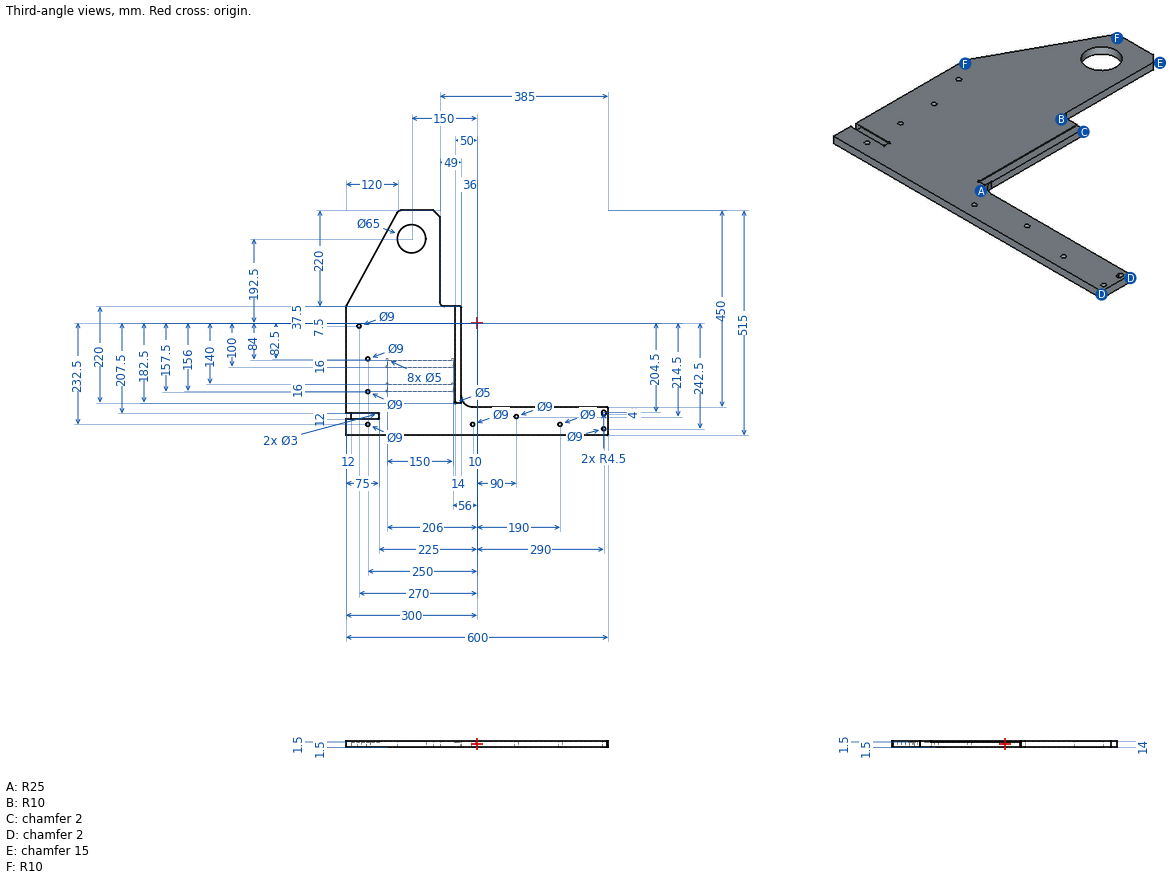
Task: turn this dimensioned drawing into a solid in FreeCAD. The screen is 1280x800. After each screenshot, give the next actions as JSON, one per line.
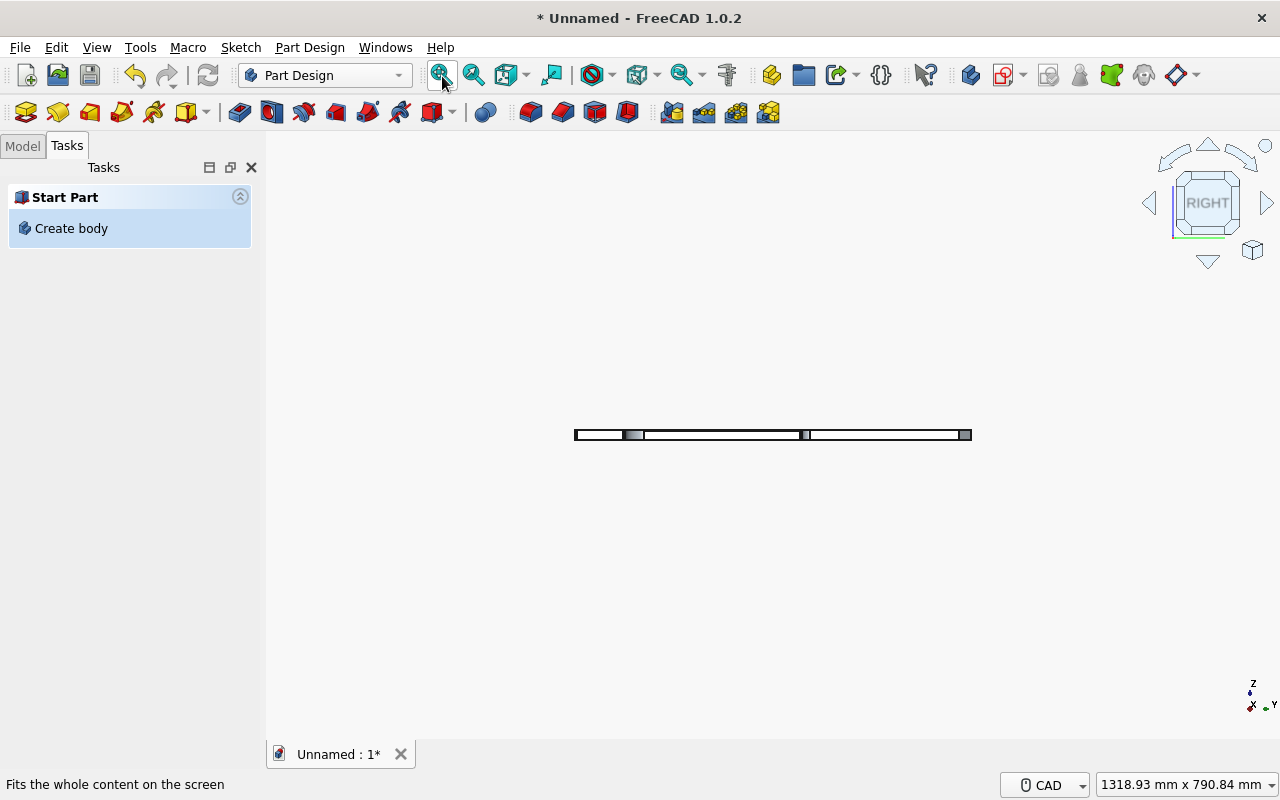
{"action": "key", "text": "5"}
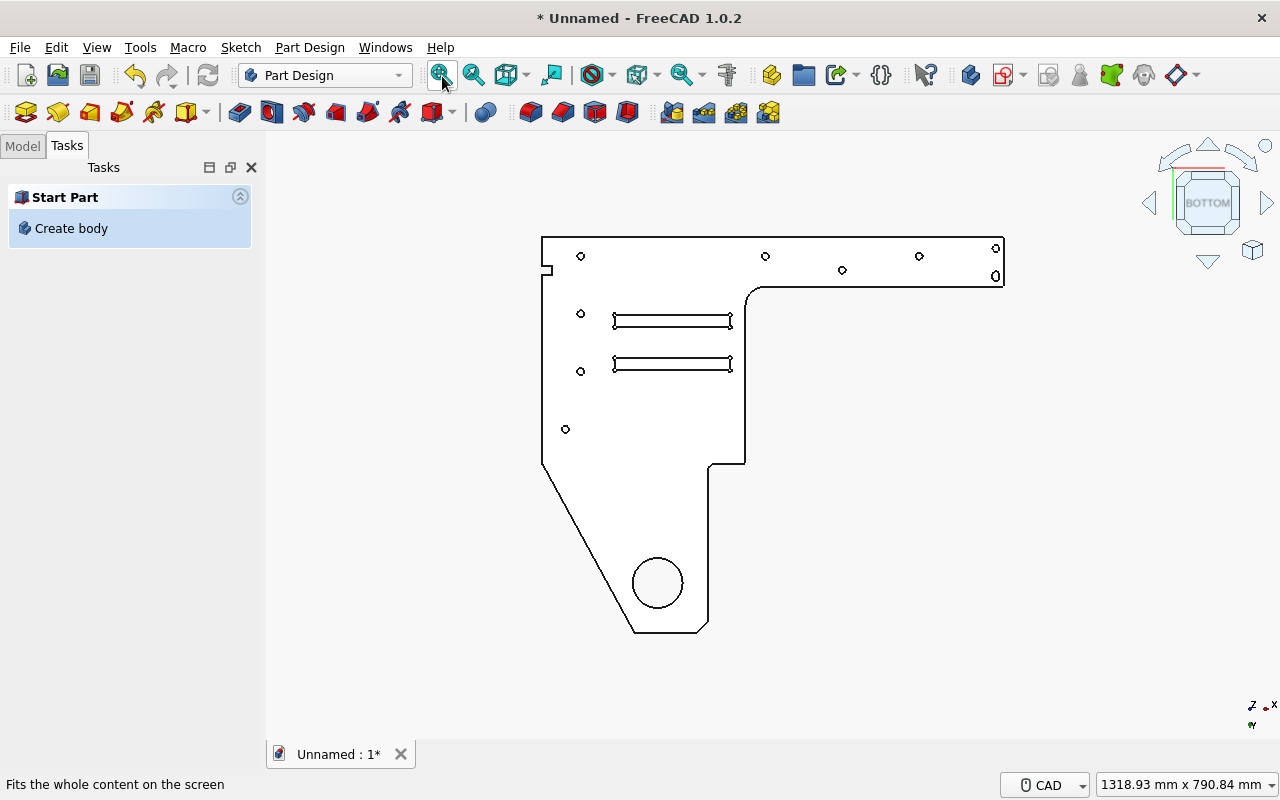
{"action": "scroll", "coordinate": [635, 632], "scroll_direction": "up", "scroll_amount": 7}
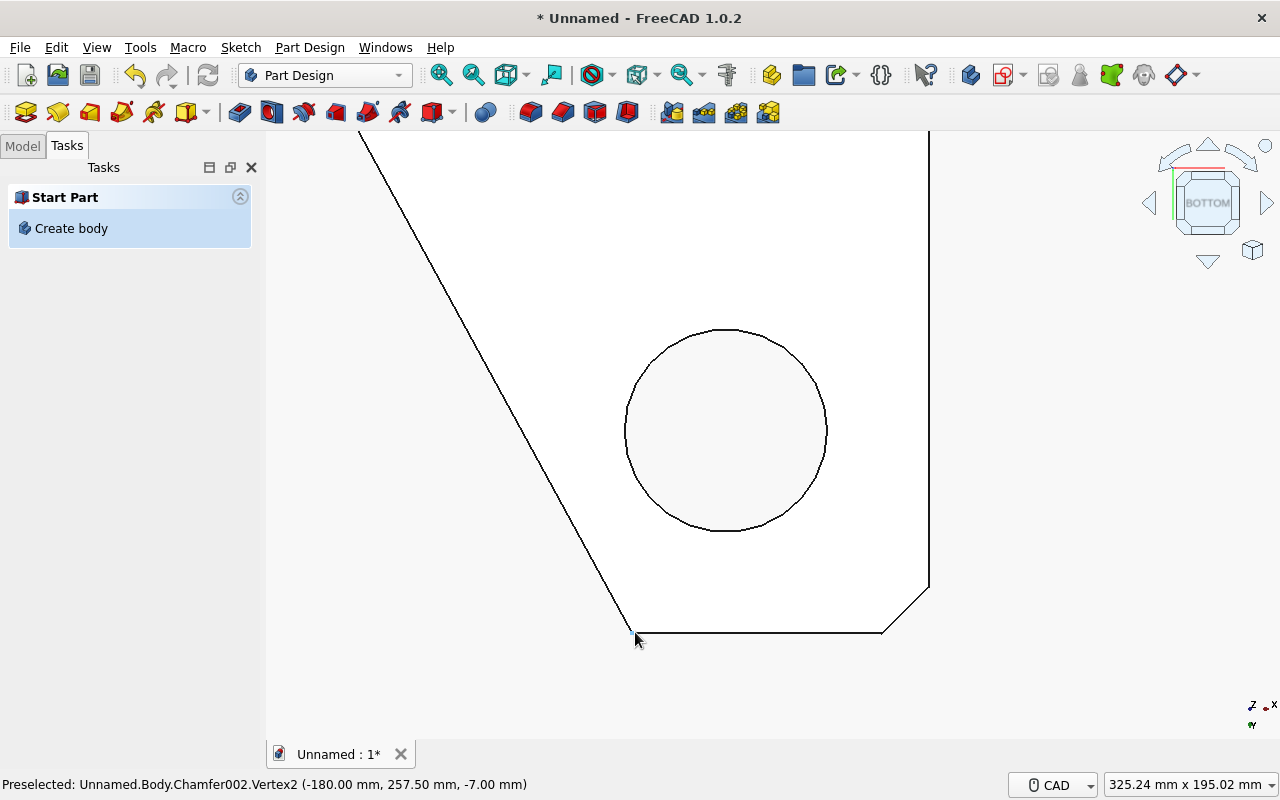
{"action": "left_click", "coordinate": [442, 76]}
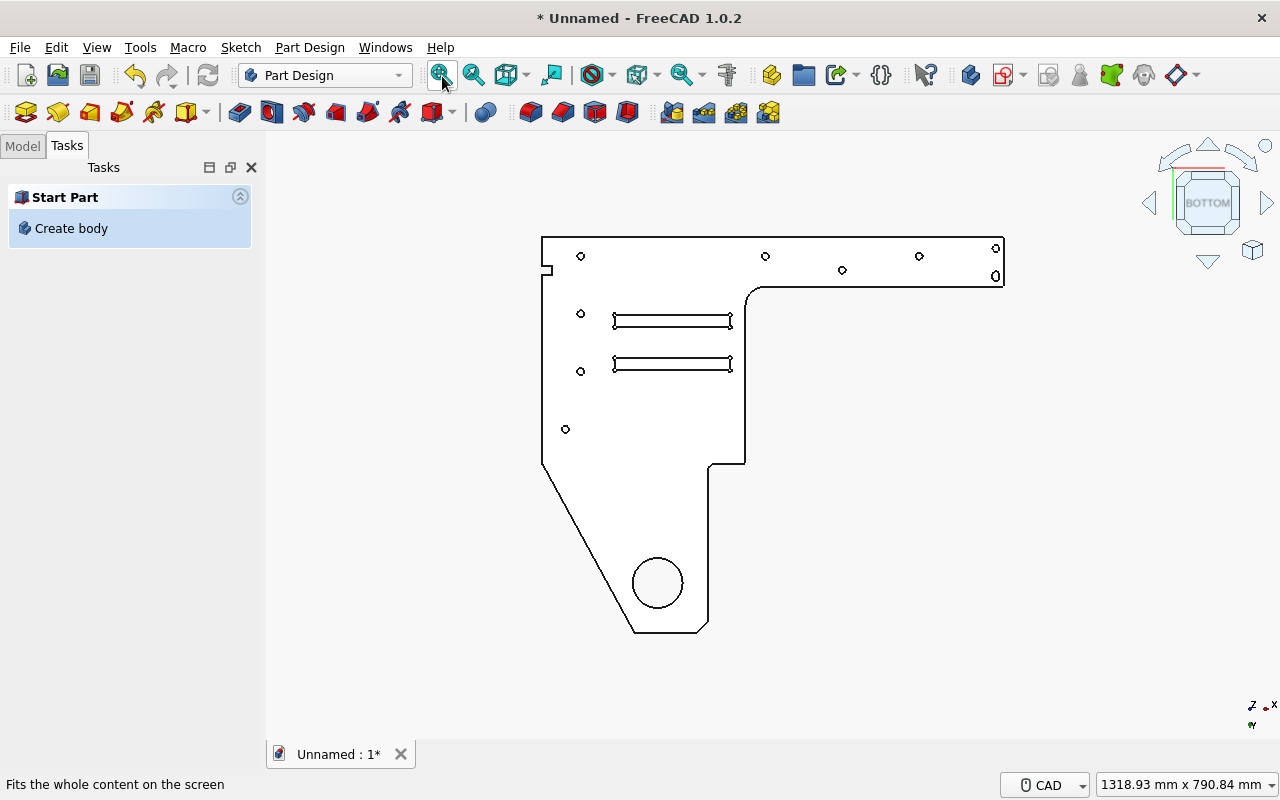
{"action": "key", "text": "4"}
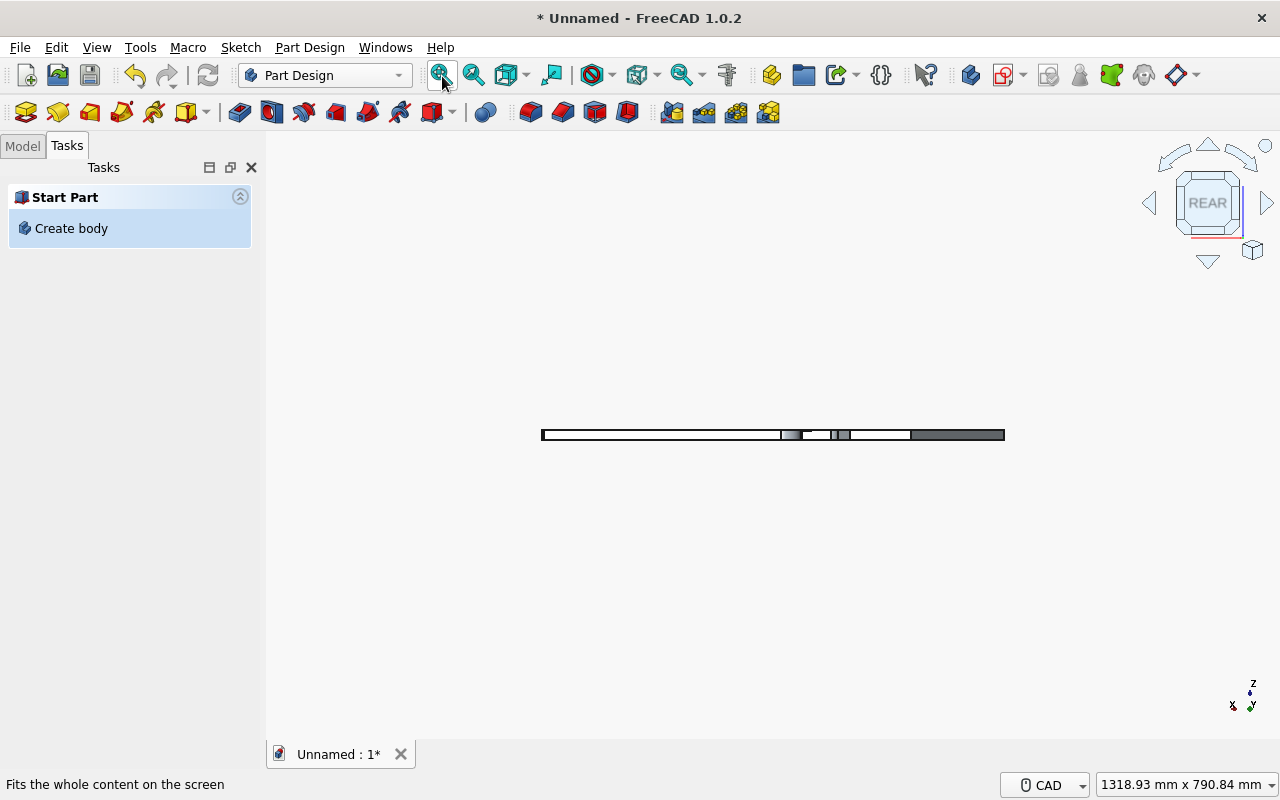
{"action": "scroll", "coordinate": [911, 434], "scroll_direction": "up", "scroll_amount": 7}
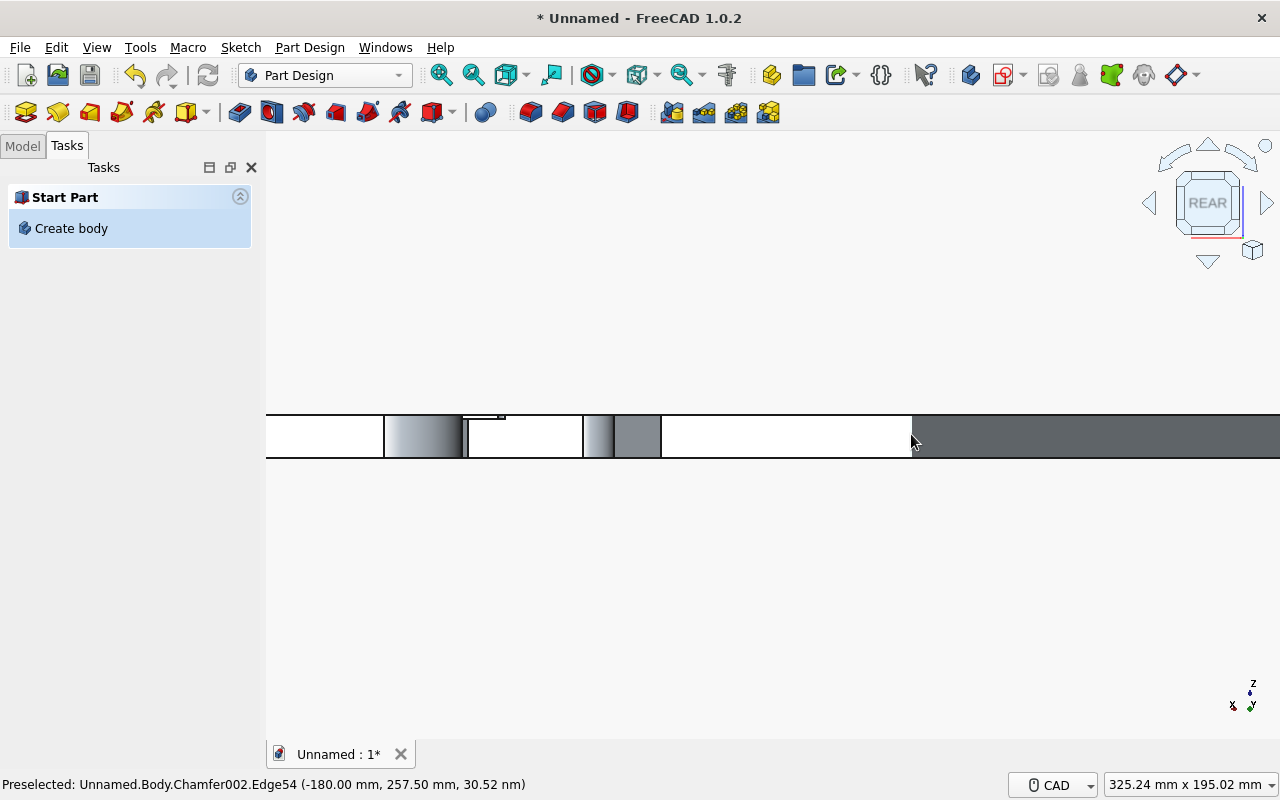
{"action": "left_click", "coordinate": [911, 436]}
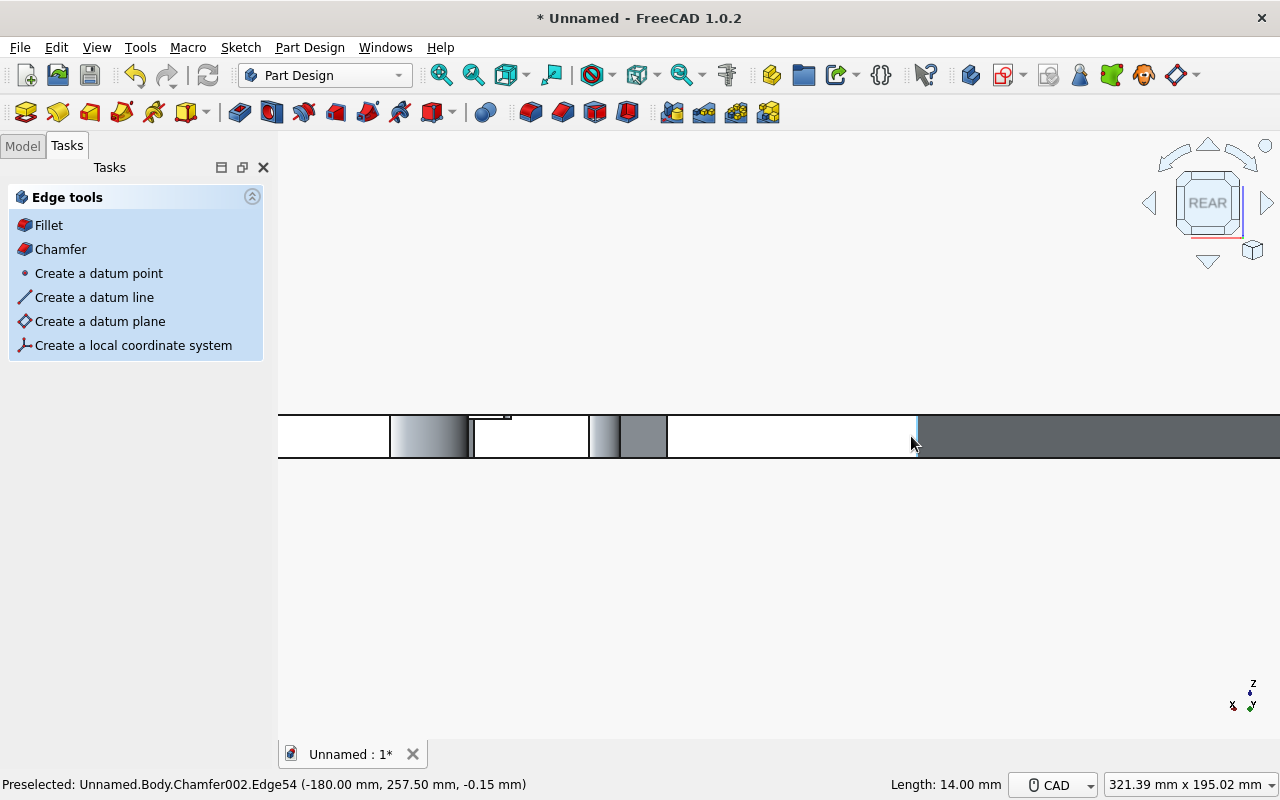
{"action": "left_click", "coordinate": [442, 76]}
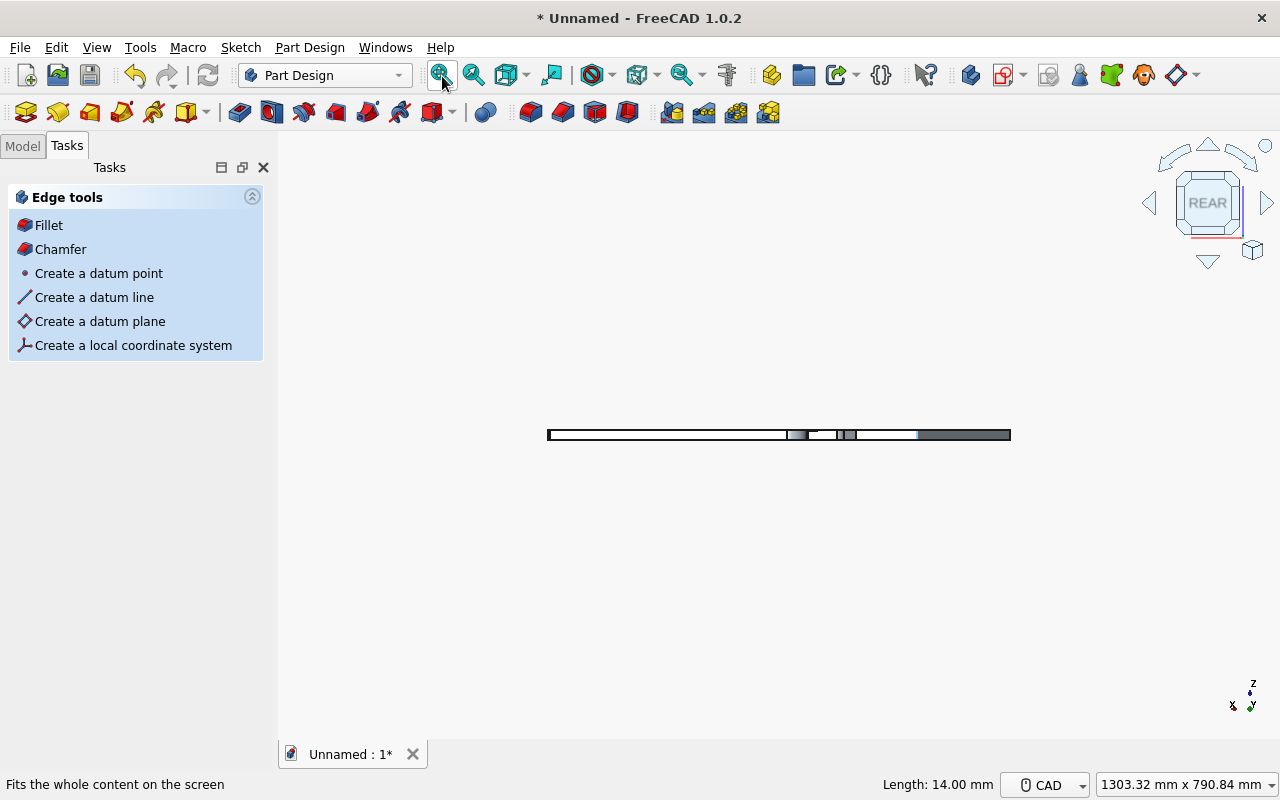
{"action": "key", "text": "6"}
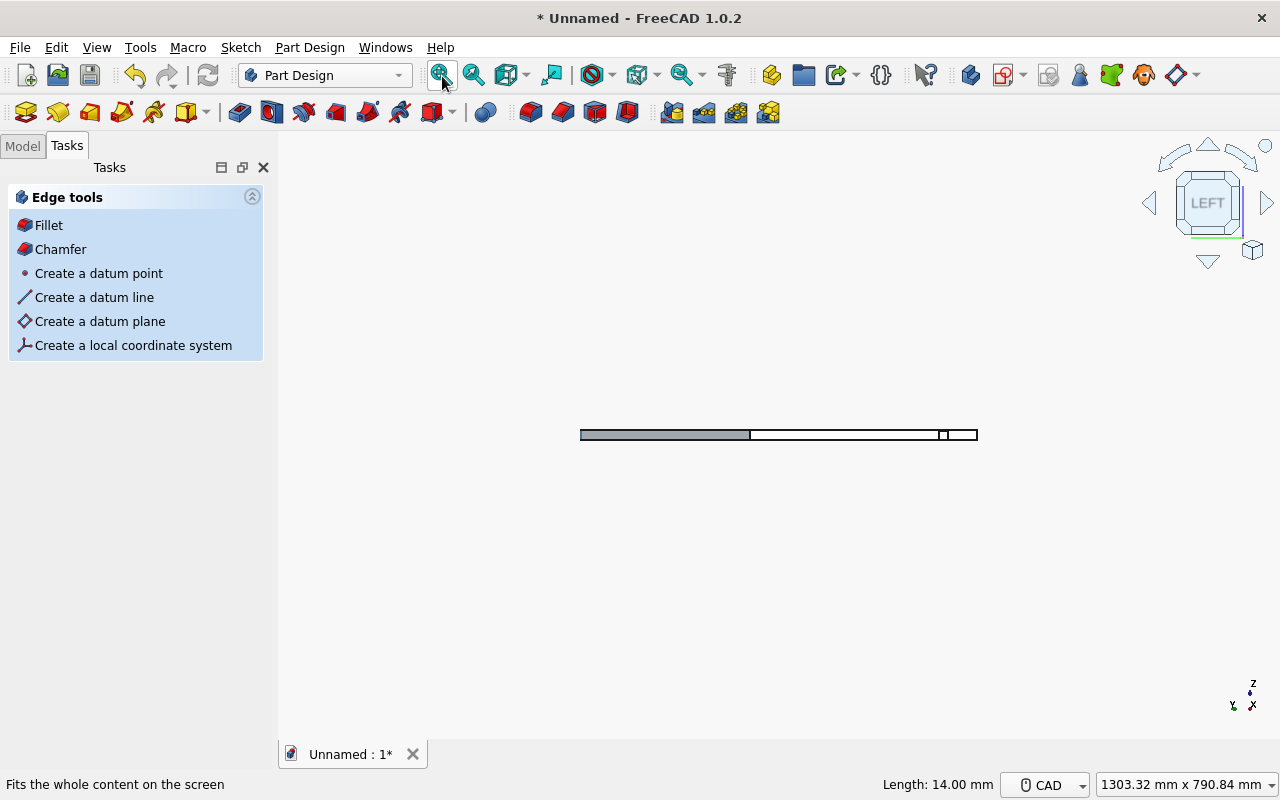
{"action": "left_click", "coordinate": [442, 76]}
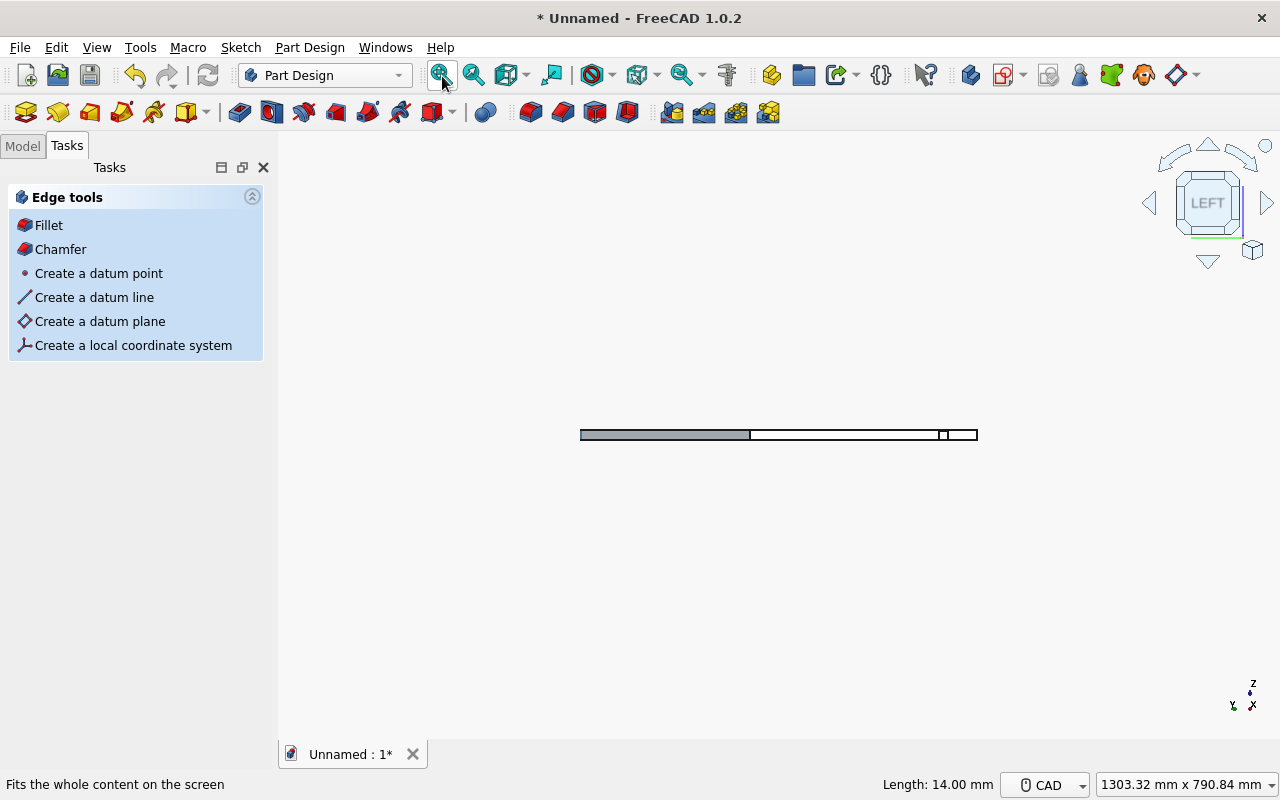
{"action": "scroll", "coordinate": [750, 434], "scroll_direction": "up", "scroll_amount": 7}